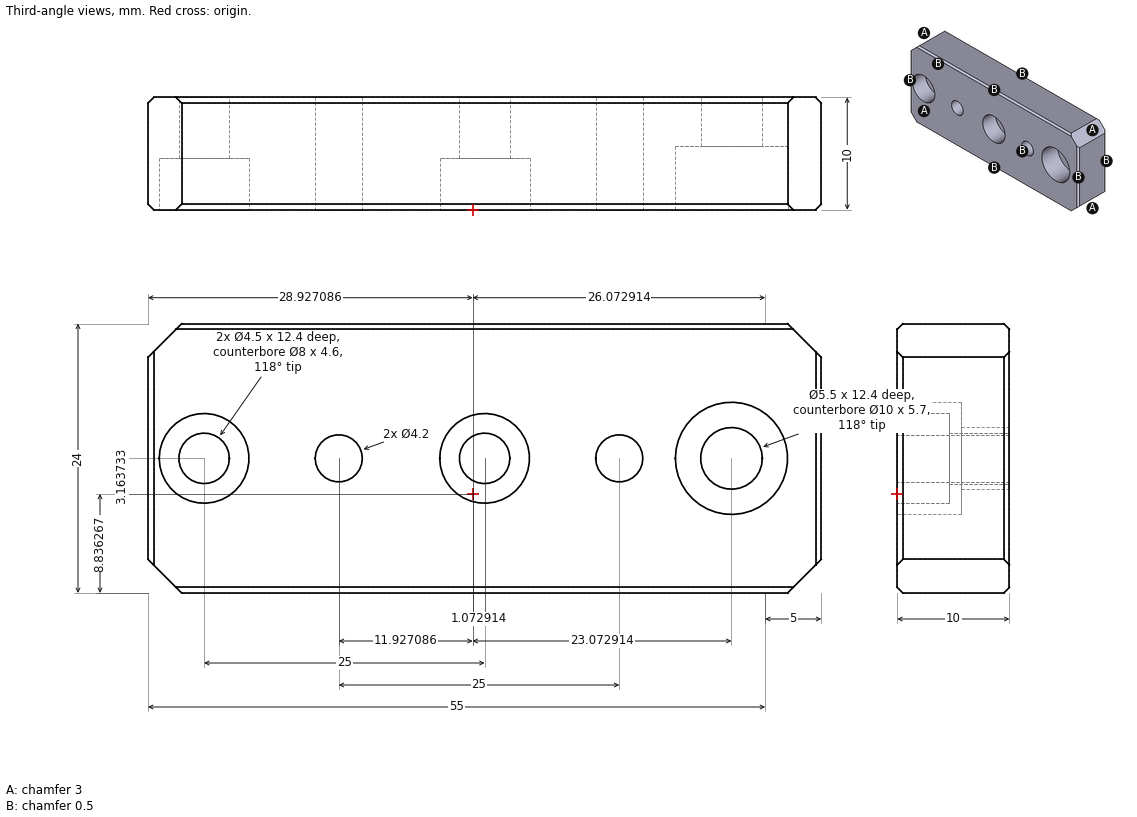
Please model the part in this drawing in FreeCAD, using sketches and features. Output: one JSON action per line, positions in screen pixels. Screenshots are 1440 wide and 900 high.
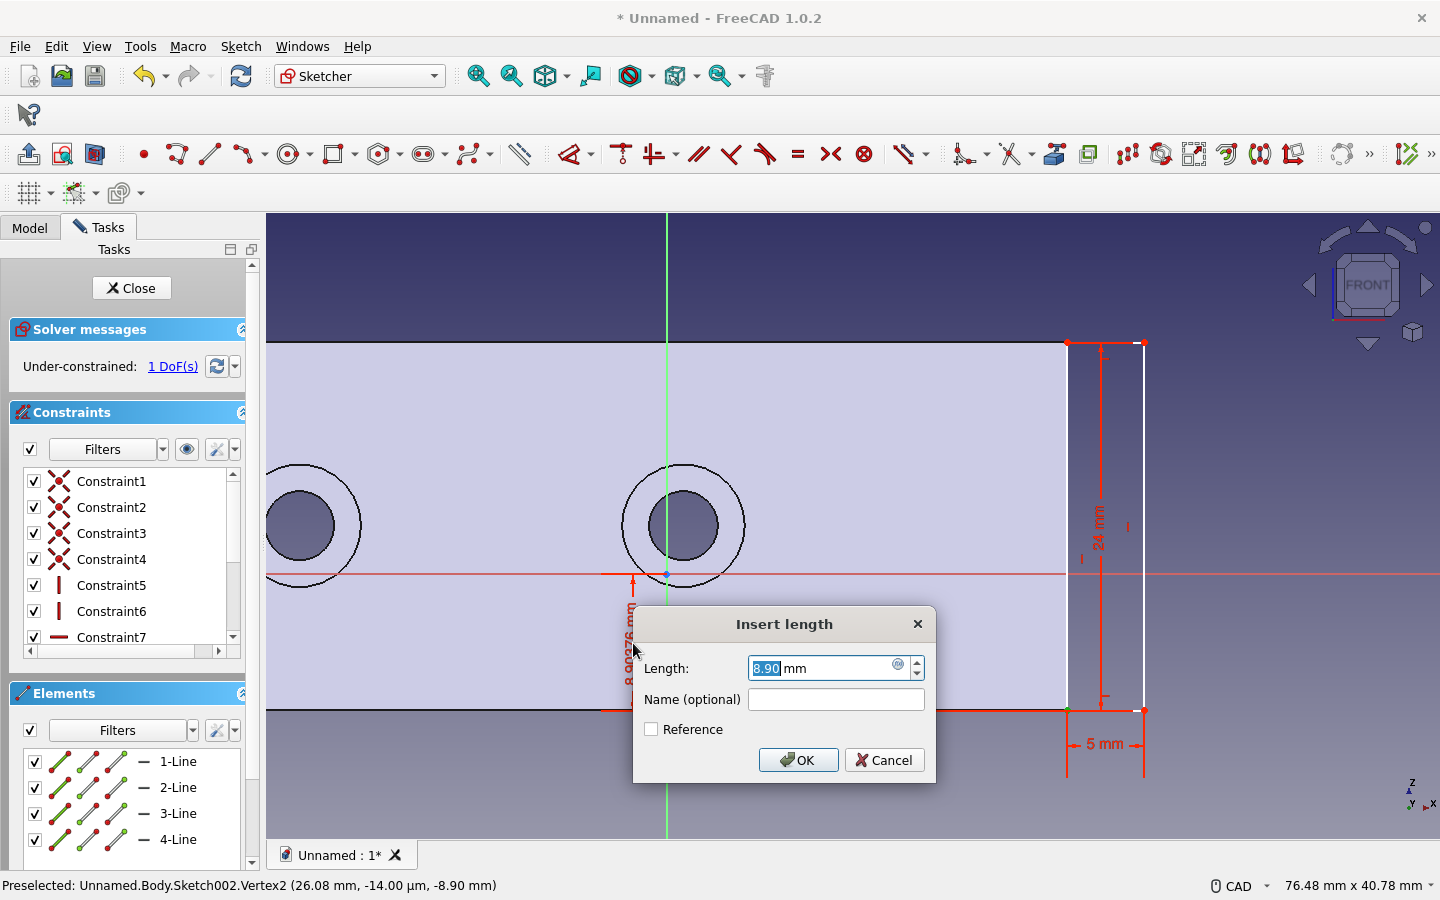
{"action": "type", "text": "8.836267"}
{"action": "key", "text": "Return"}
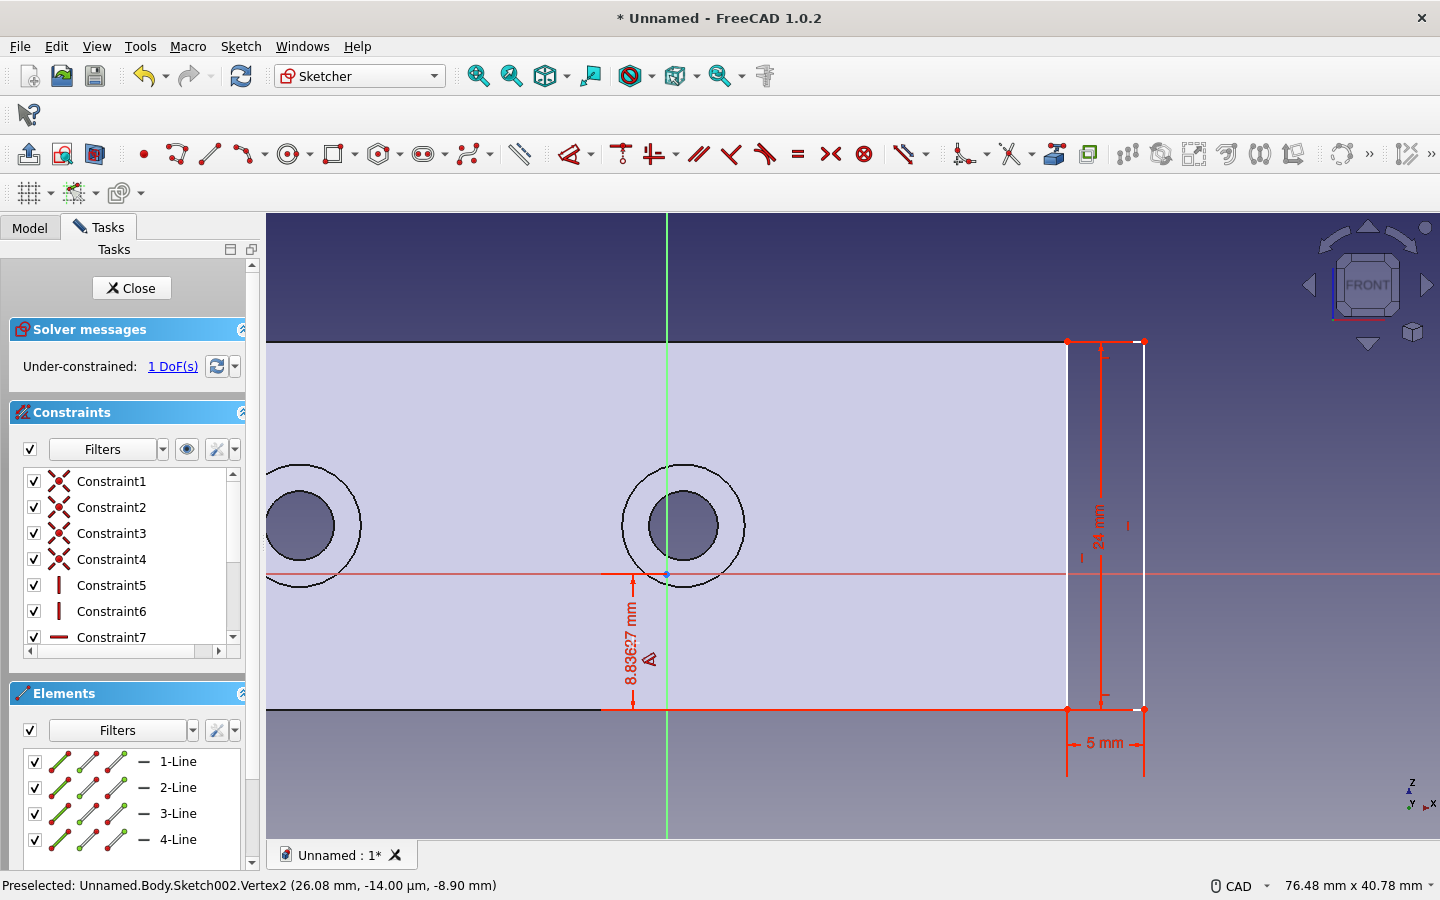
{"action": "left_click", "coordinate": [1067, 342]}
{"action": "left_click", "coordinate": [867, 308]}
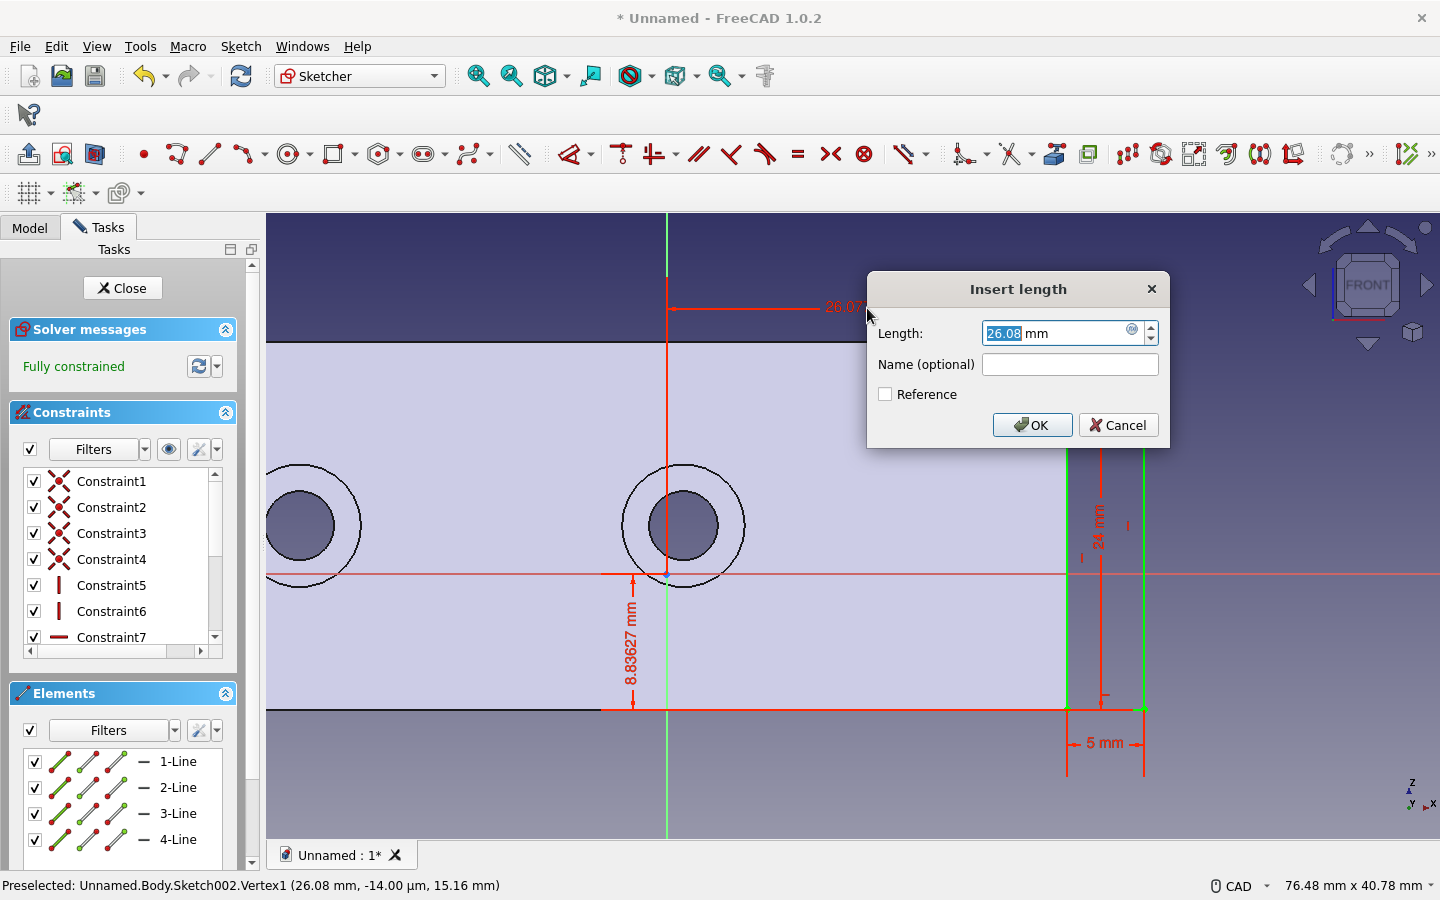
{"action": "type", "text": "26.072914"}
{"action": "key", "text": "Return"}
{"action": "key", "text": "Escape"}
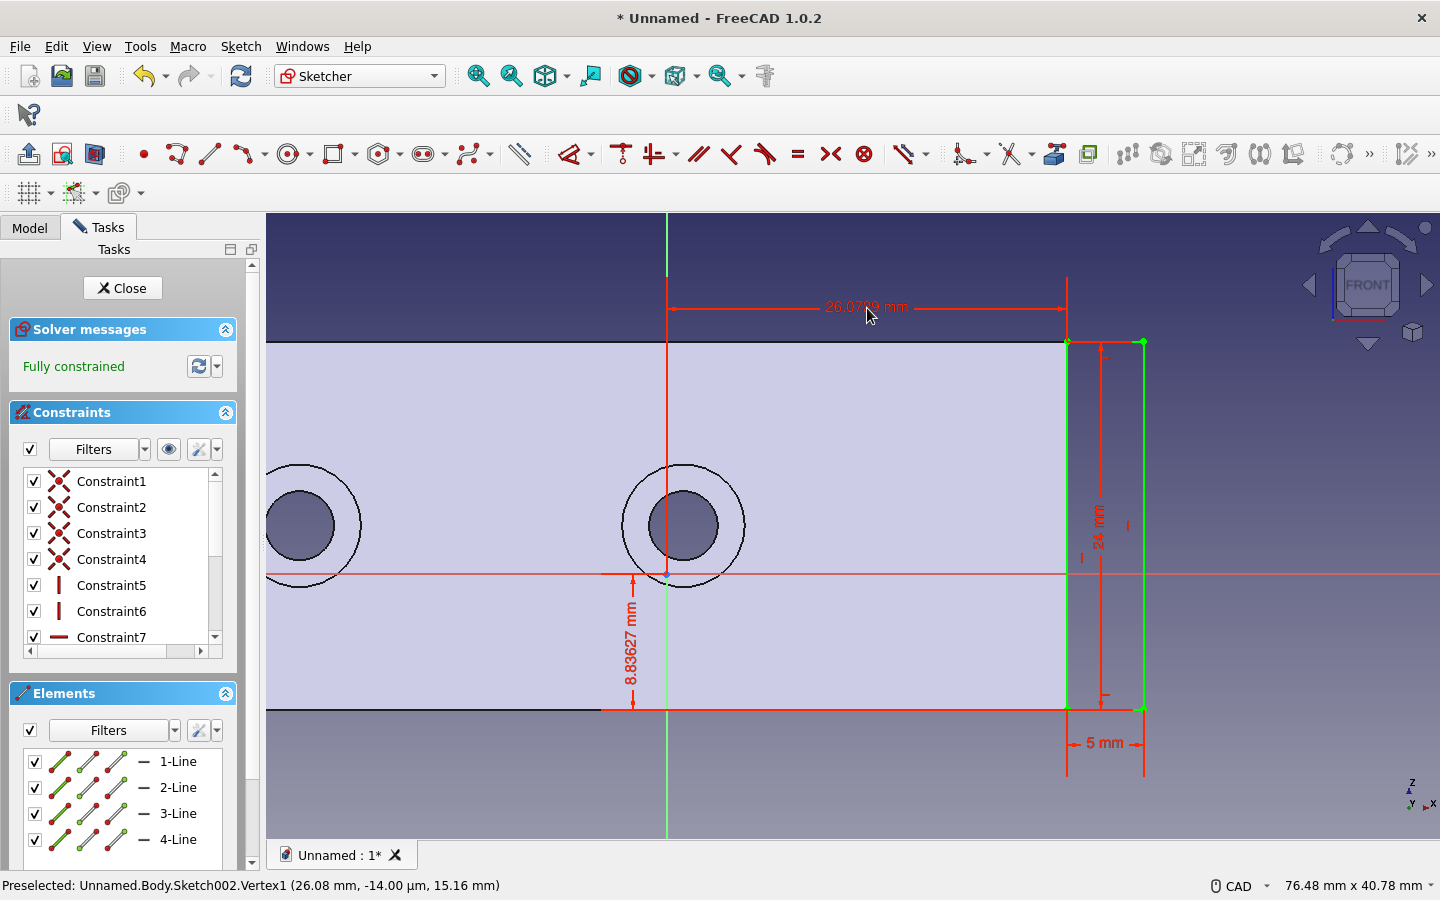
{"action": "left_click", "coordinate": [123, 288]}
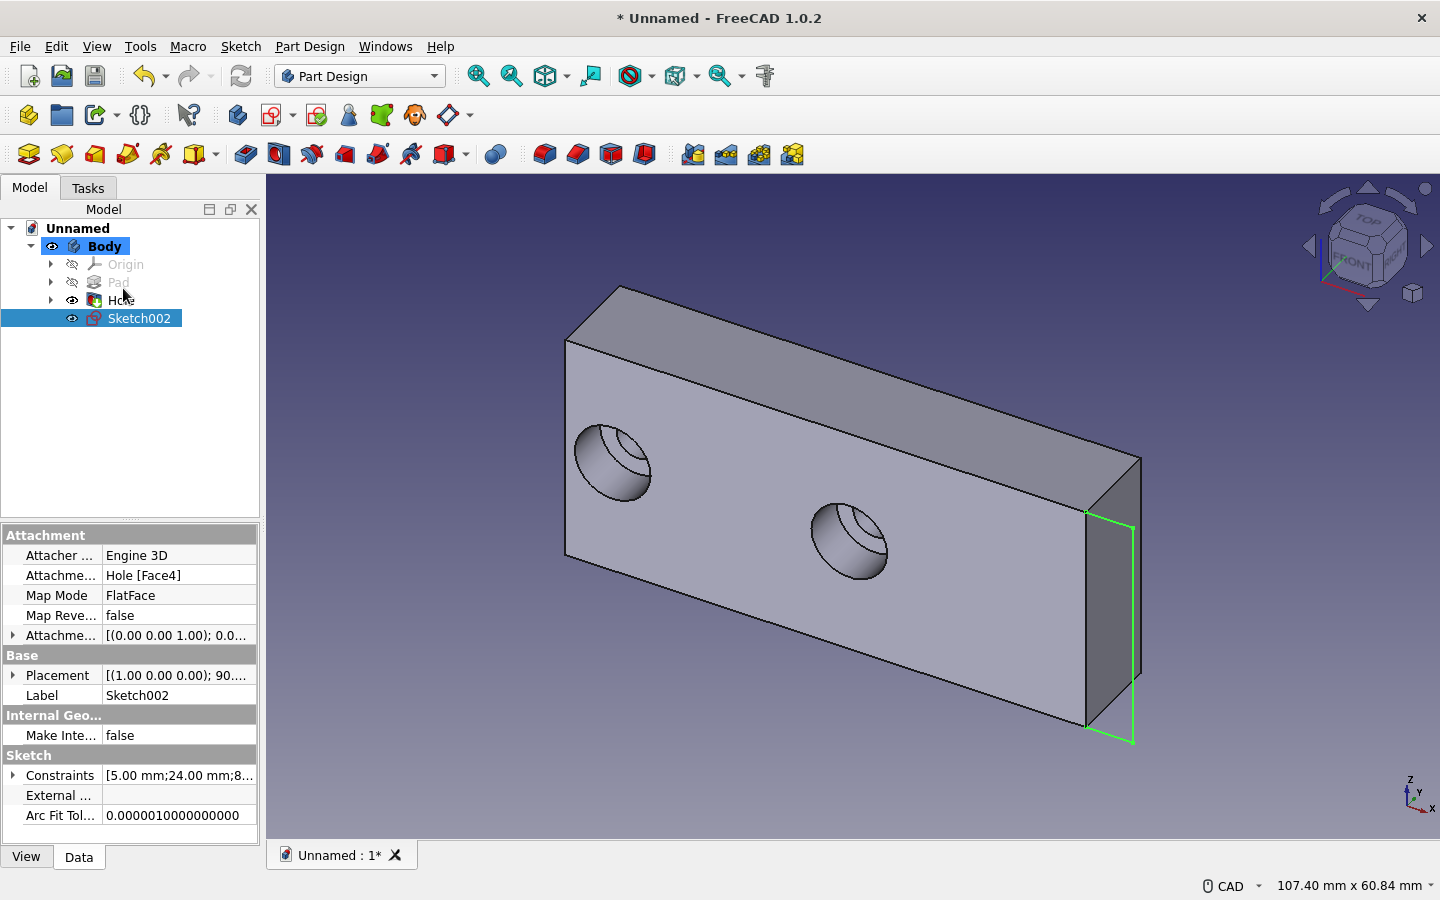
{"action": "left_click", "coordinate": [29, 154]}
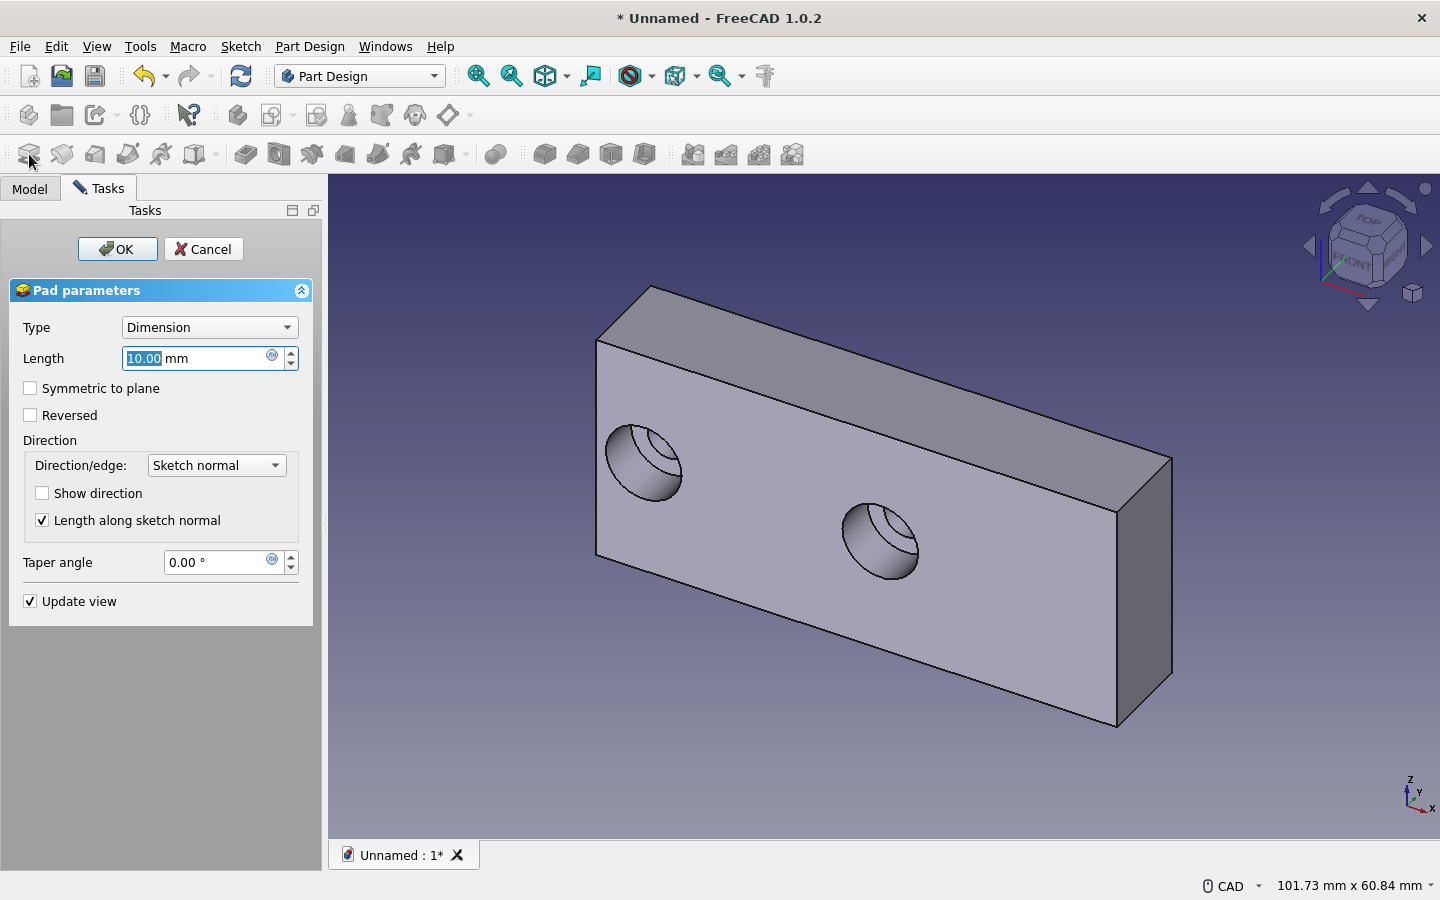
{"action": "type", "text": "10"}
{"action": "key", "text": "Tab"}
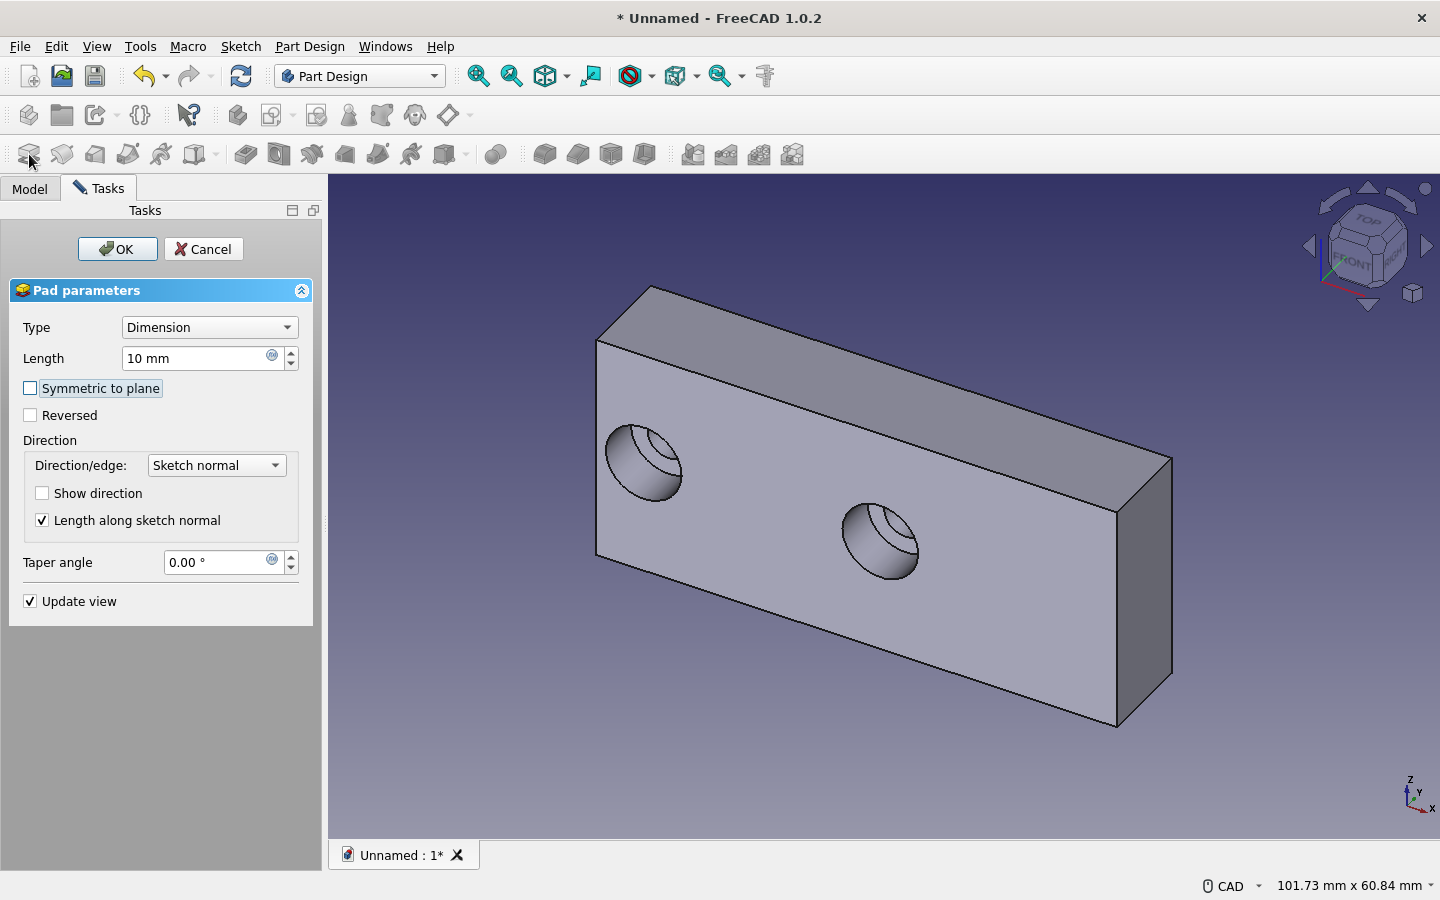
{"action": "left_click", "coordinate": [31, 415]}